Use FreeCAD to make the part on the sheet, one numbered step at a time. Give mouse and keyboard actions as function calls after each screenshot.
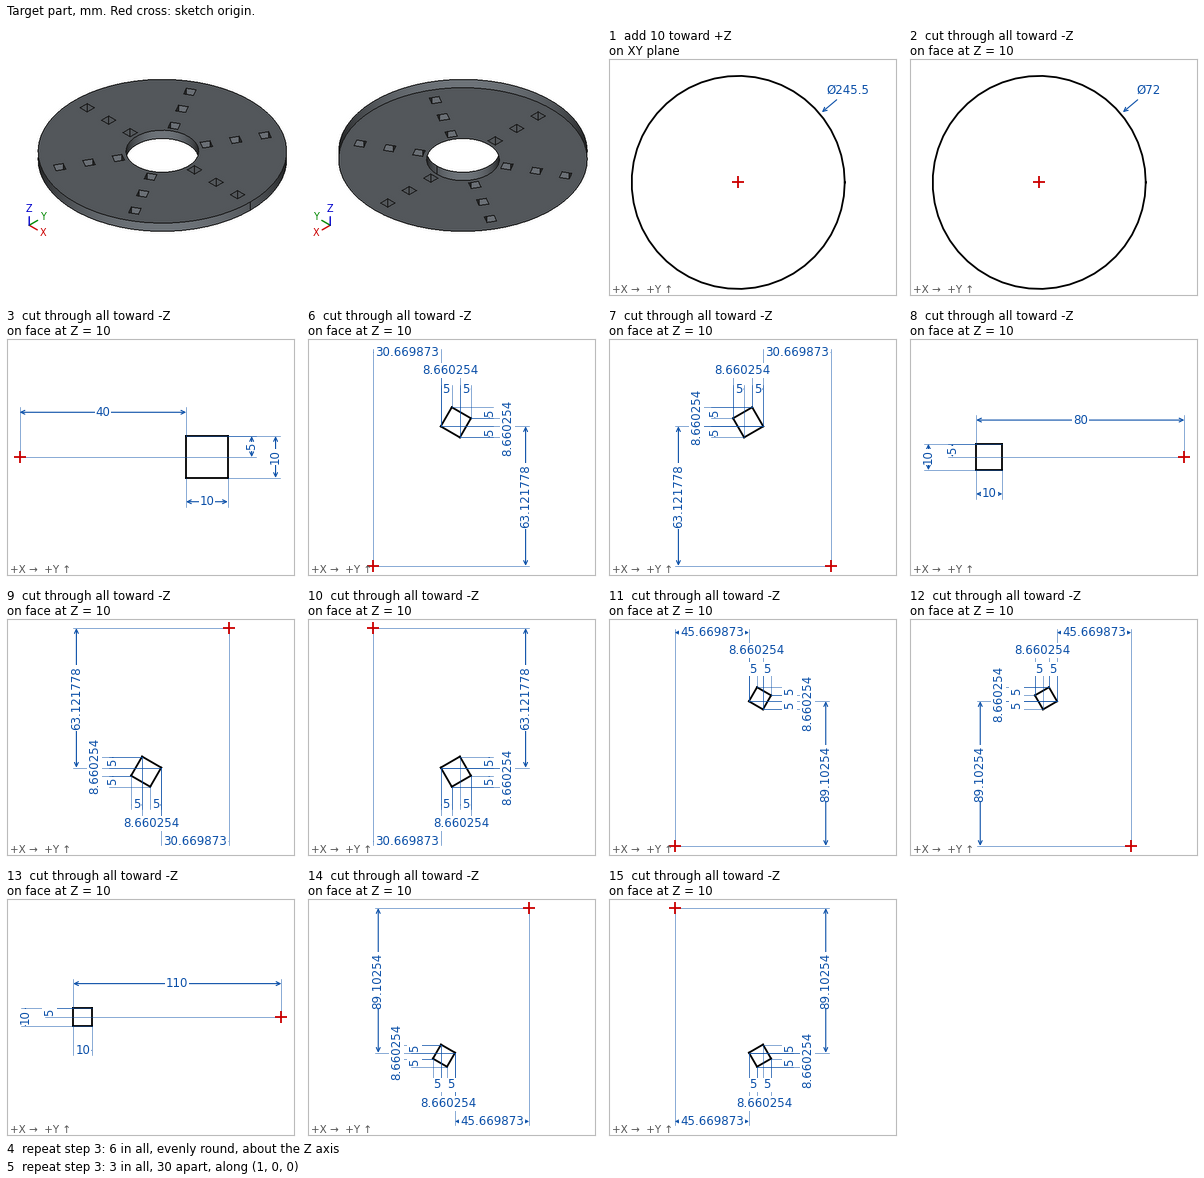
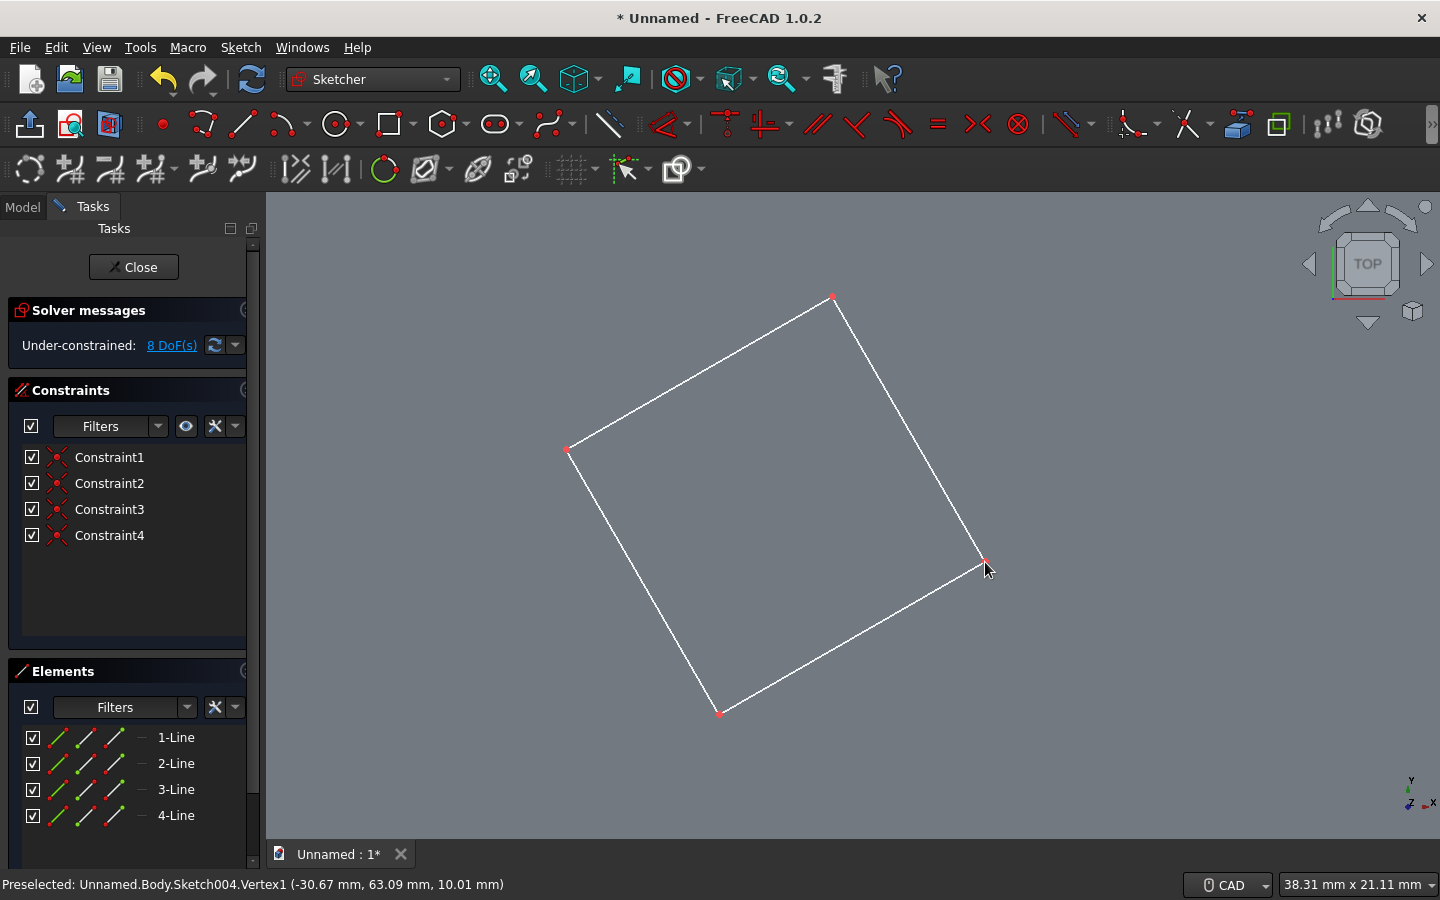
key(d)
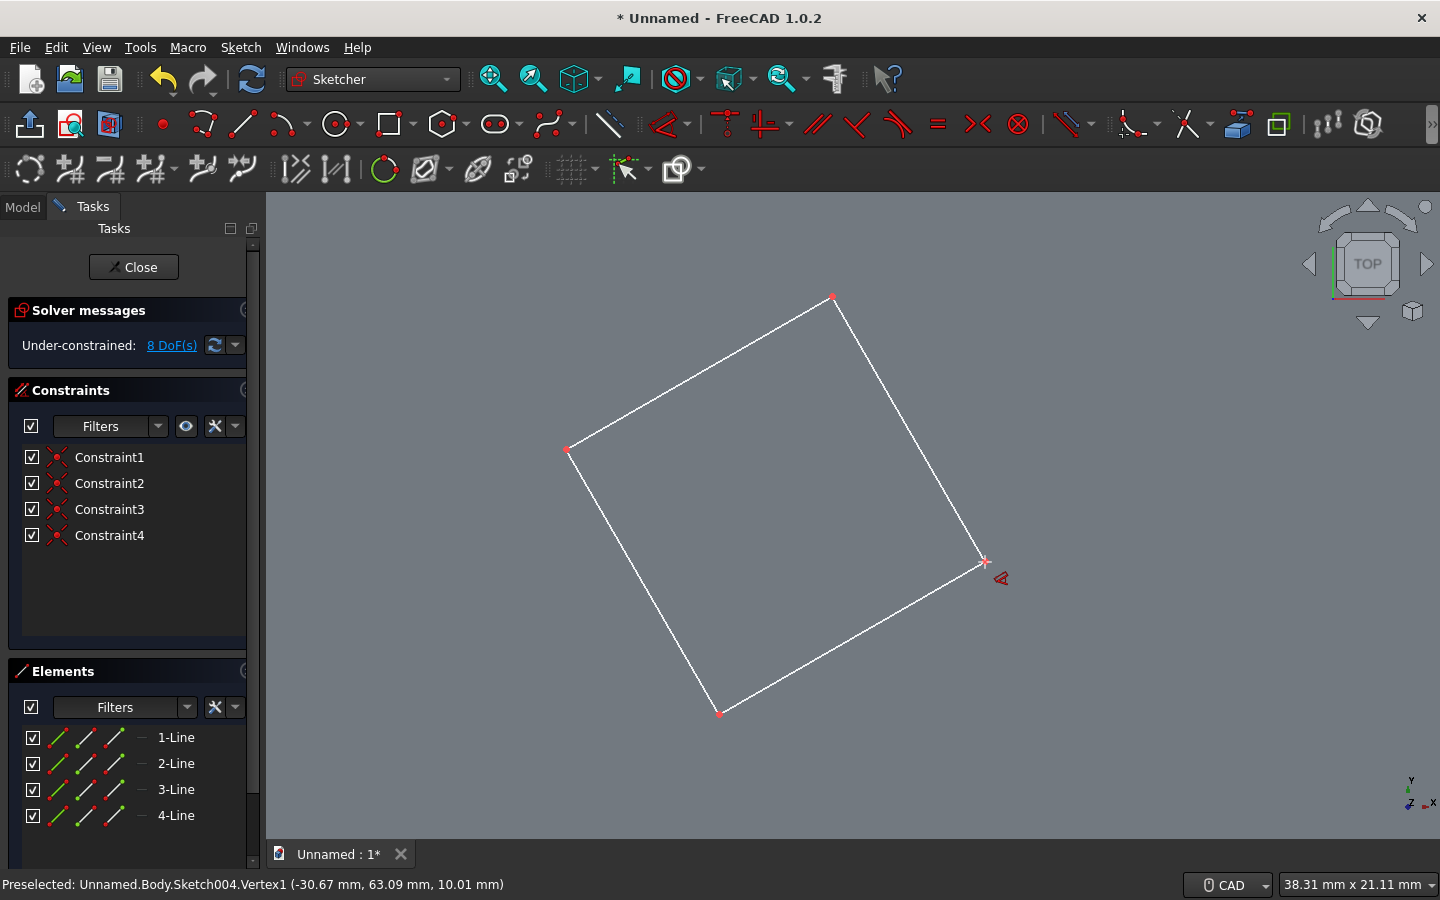
click(939, 482)
click(908, 263)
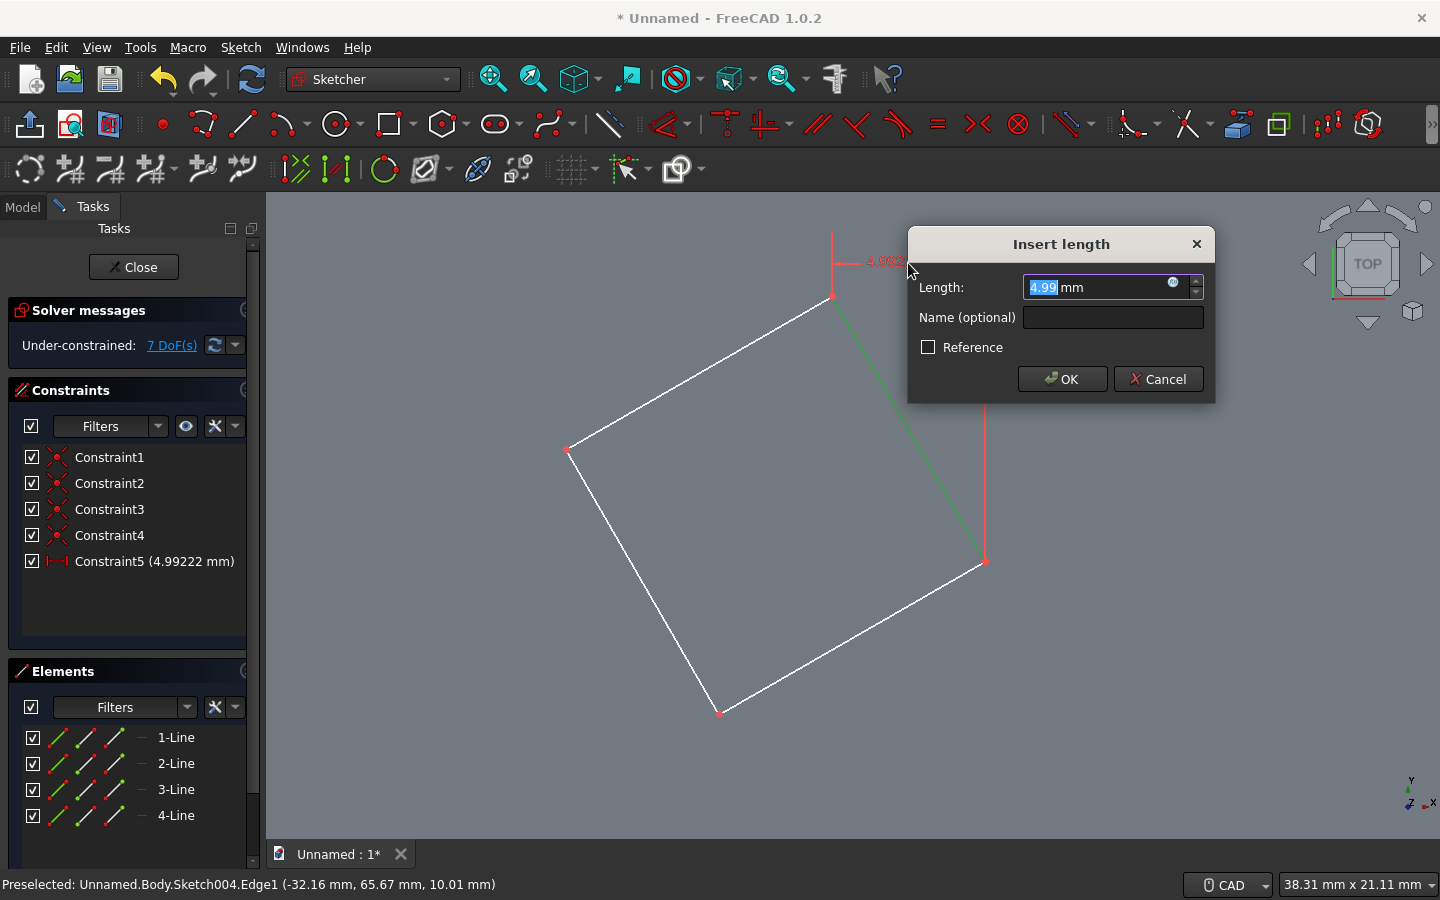
text(5)
key(Return)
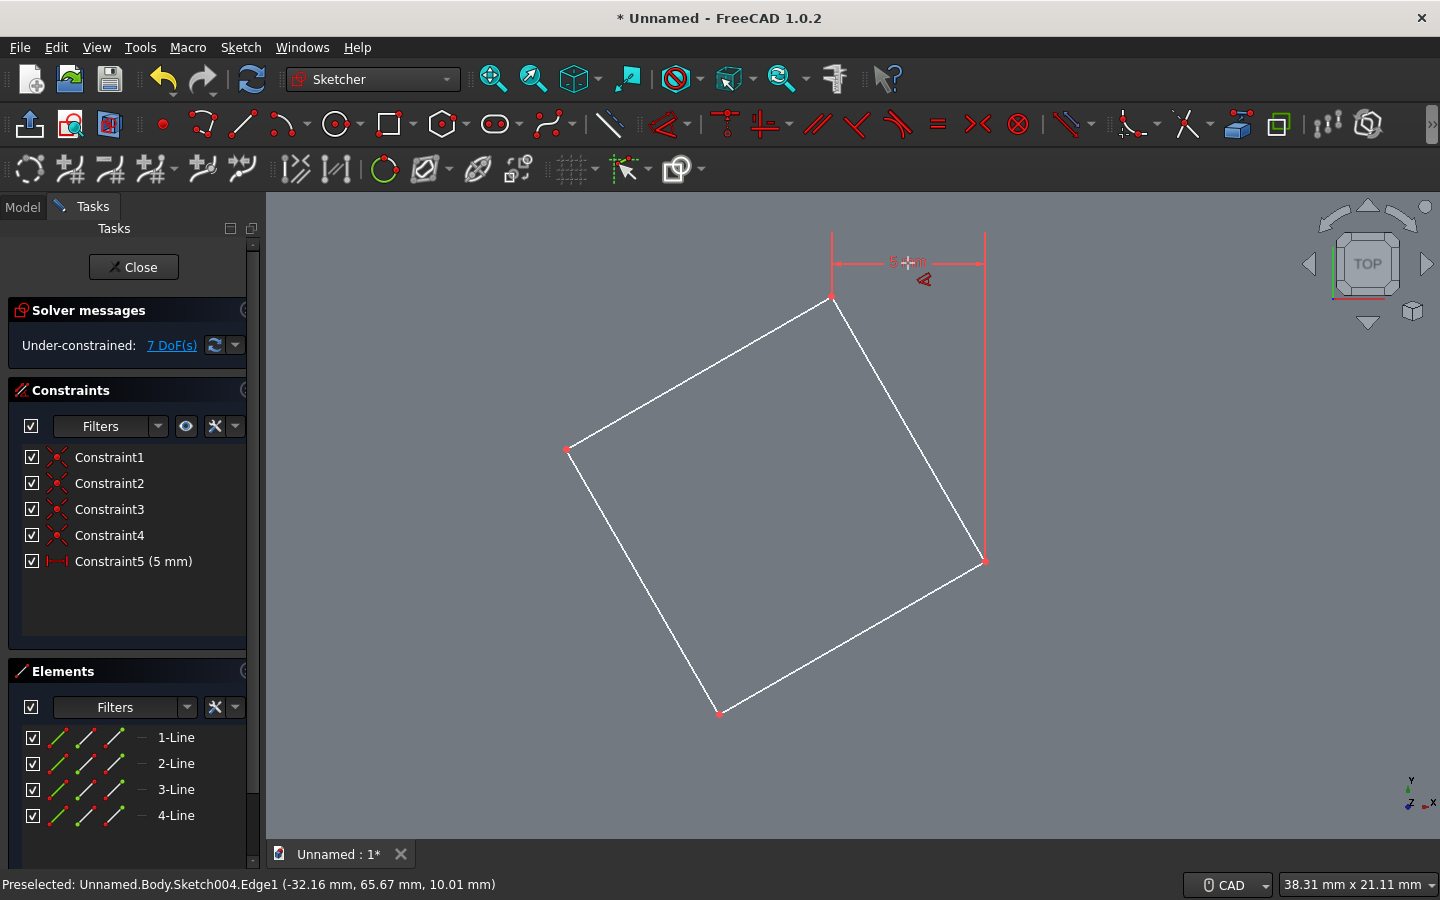
click(752, 343)
click(532, 373)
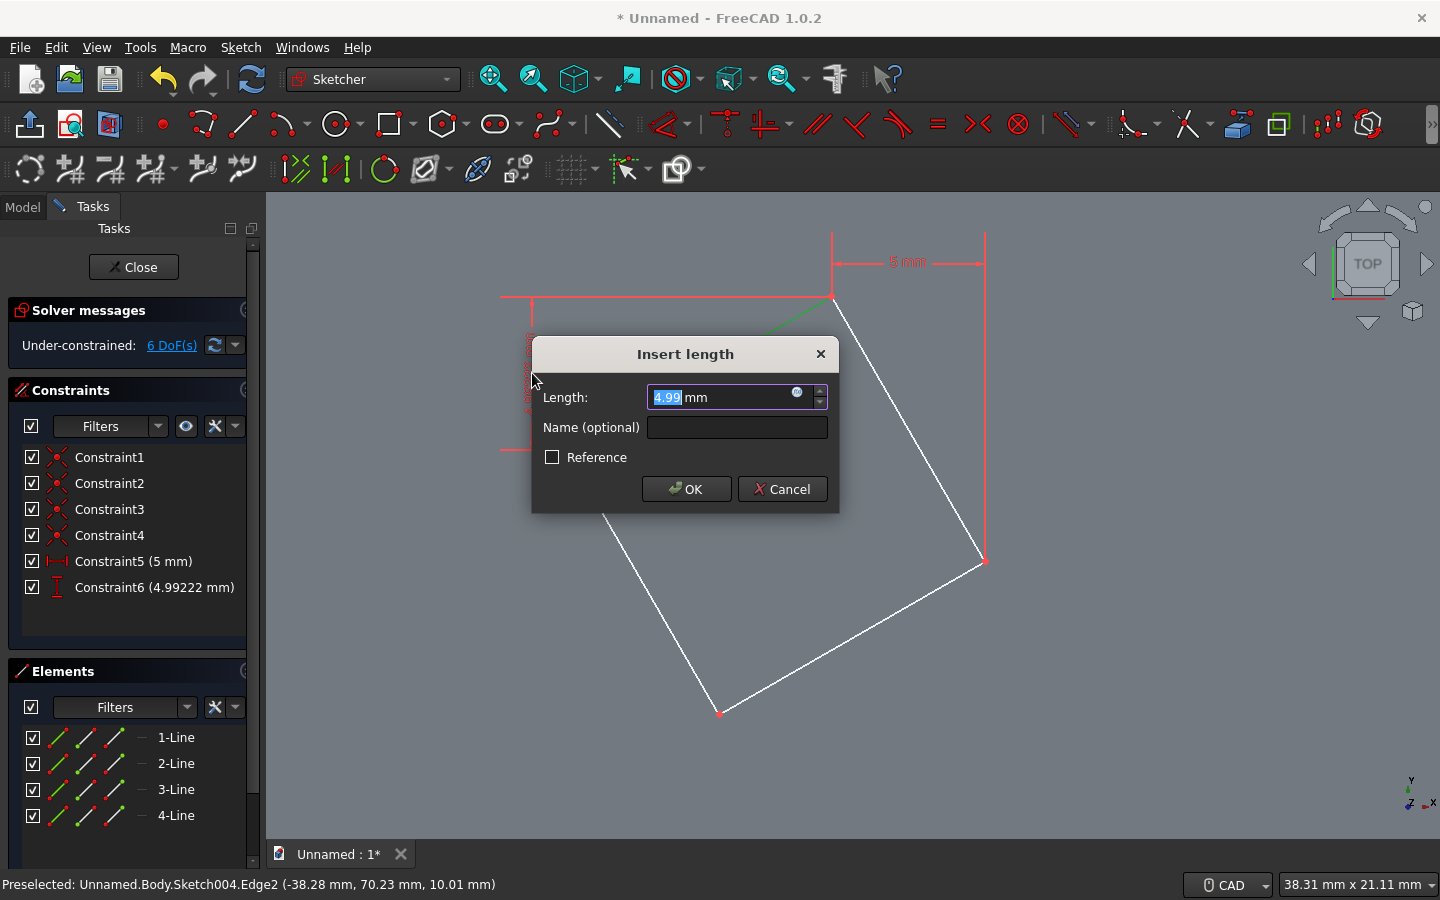
text(5)
key(Return)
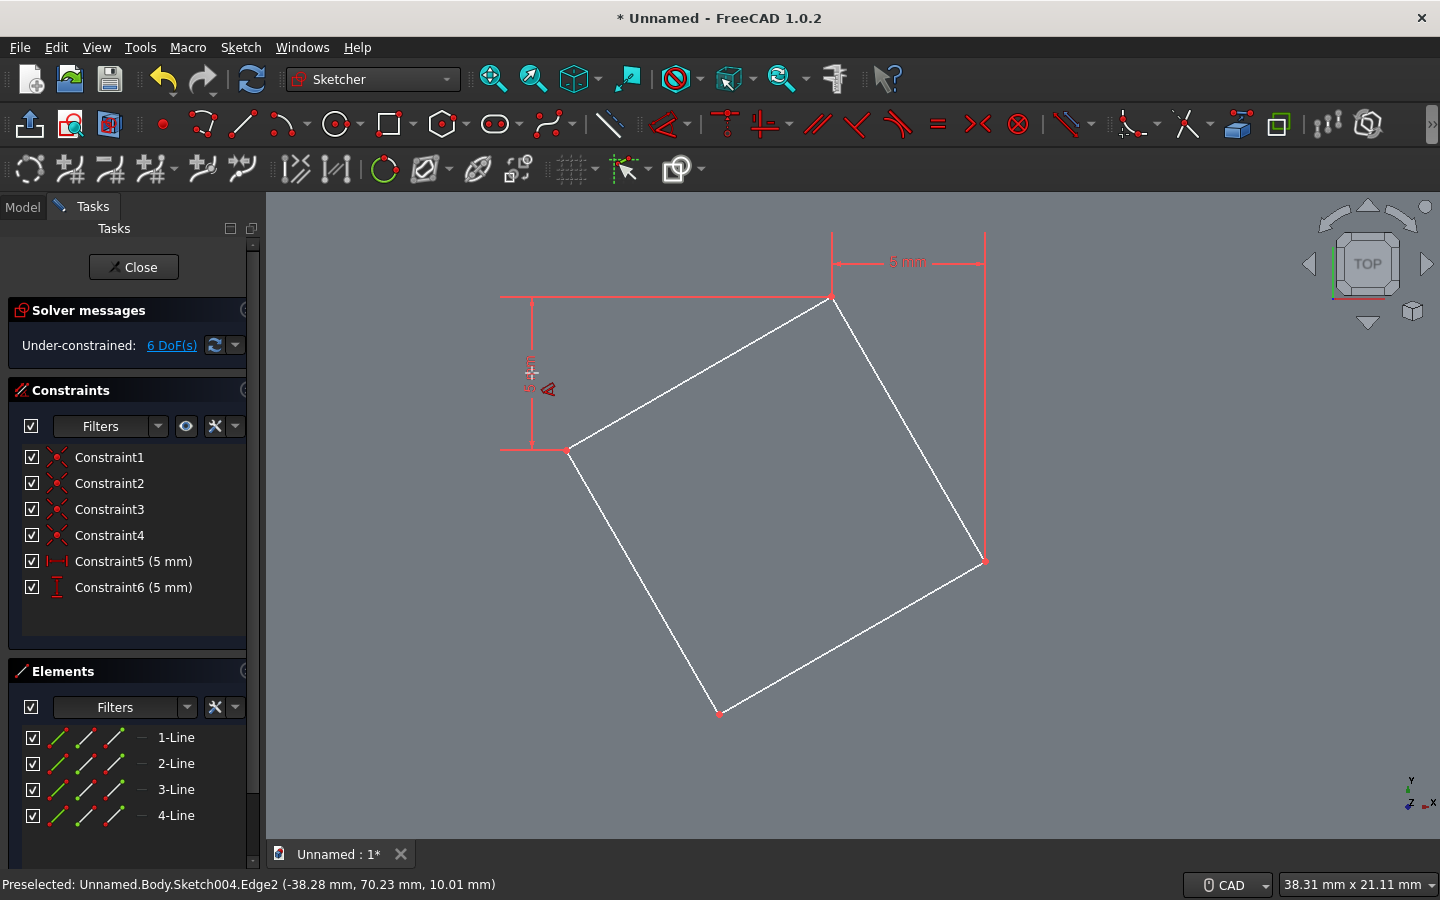
click(612, 530)
click(642, 749)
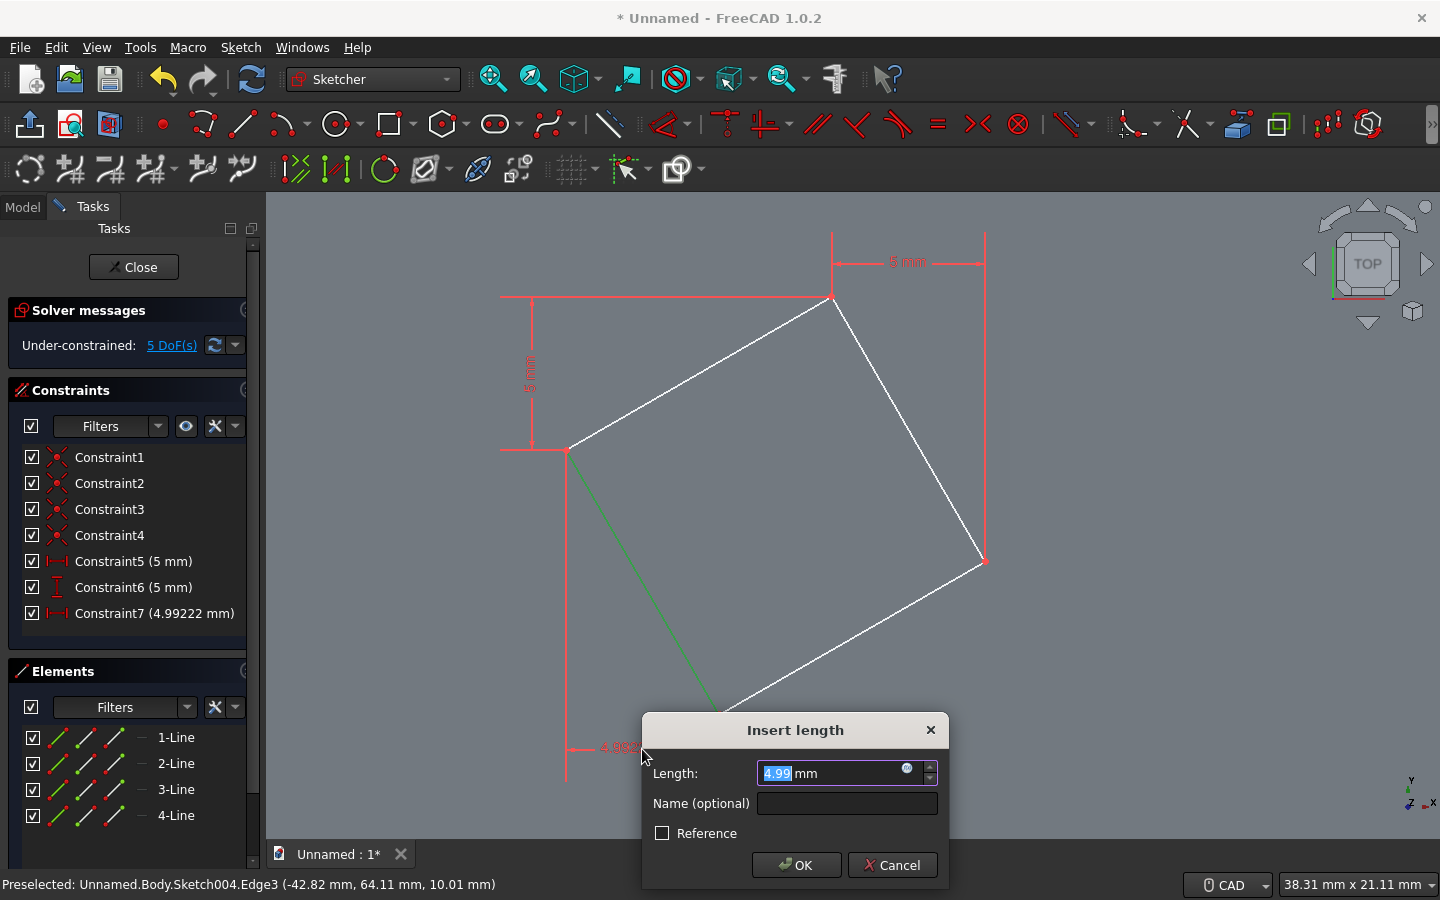
text(5)
key(Return)